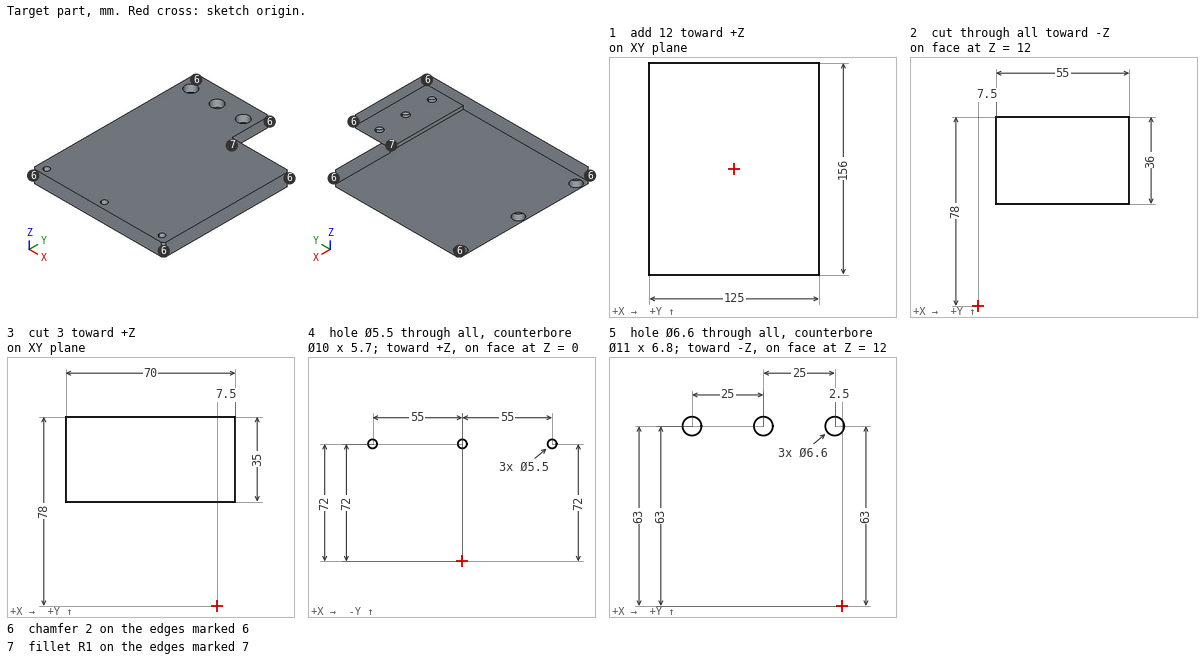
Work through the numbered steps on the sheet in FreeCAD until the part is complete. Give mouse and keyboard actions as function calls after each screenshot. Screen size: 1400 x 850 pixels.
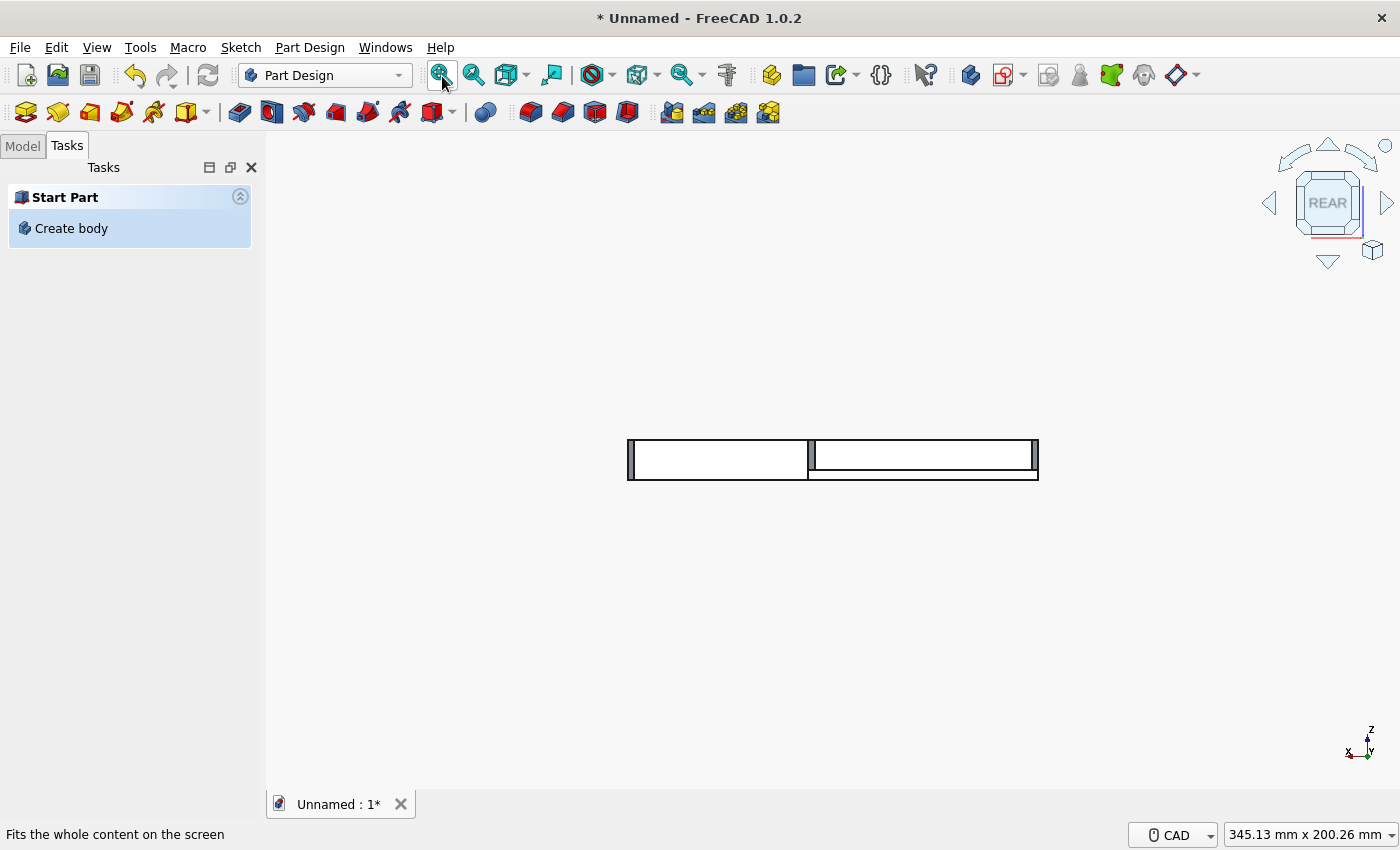
key(0)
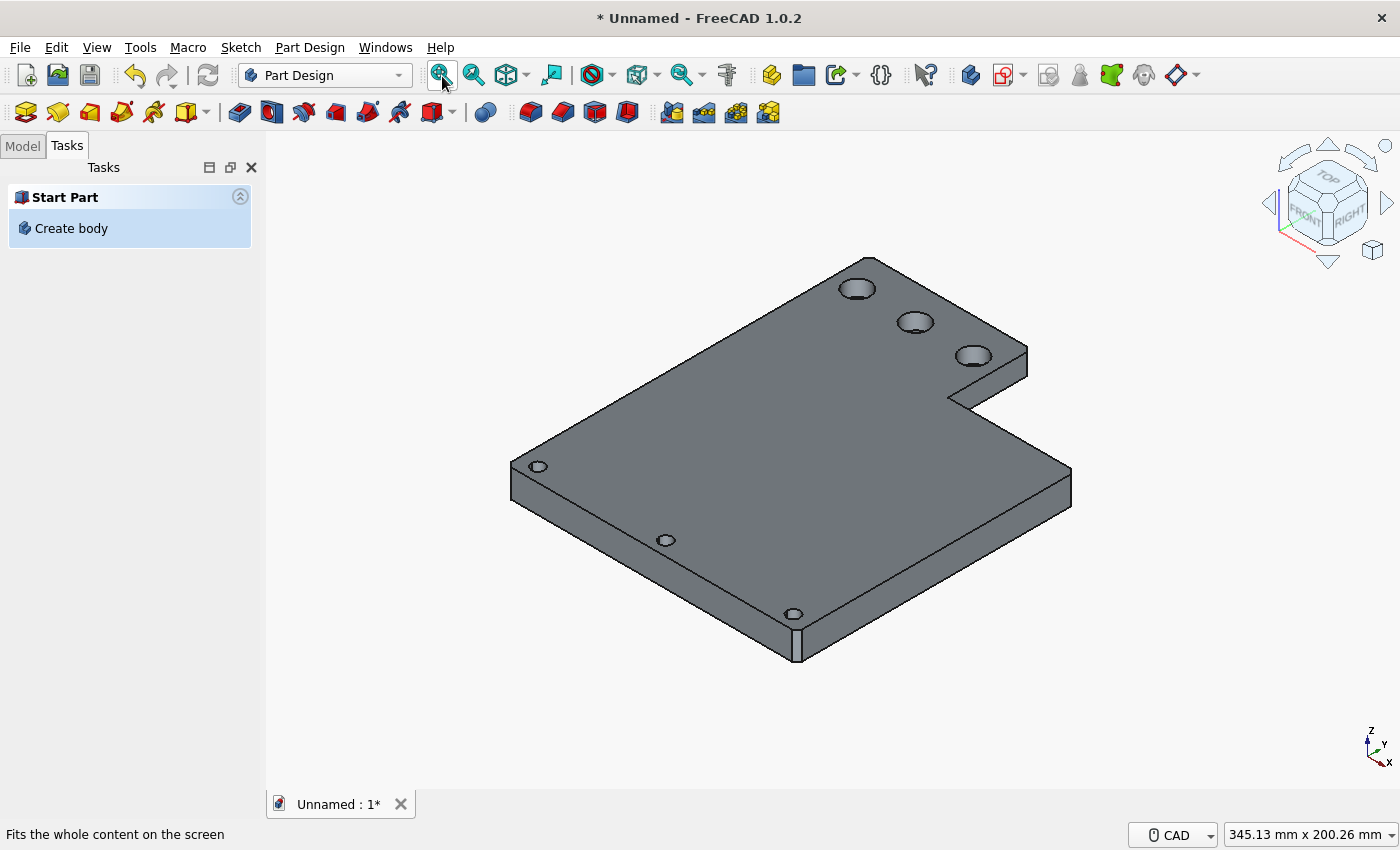
key(2)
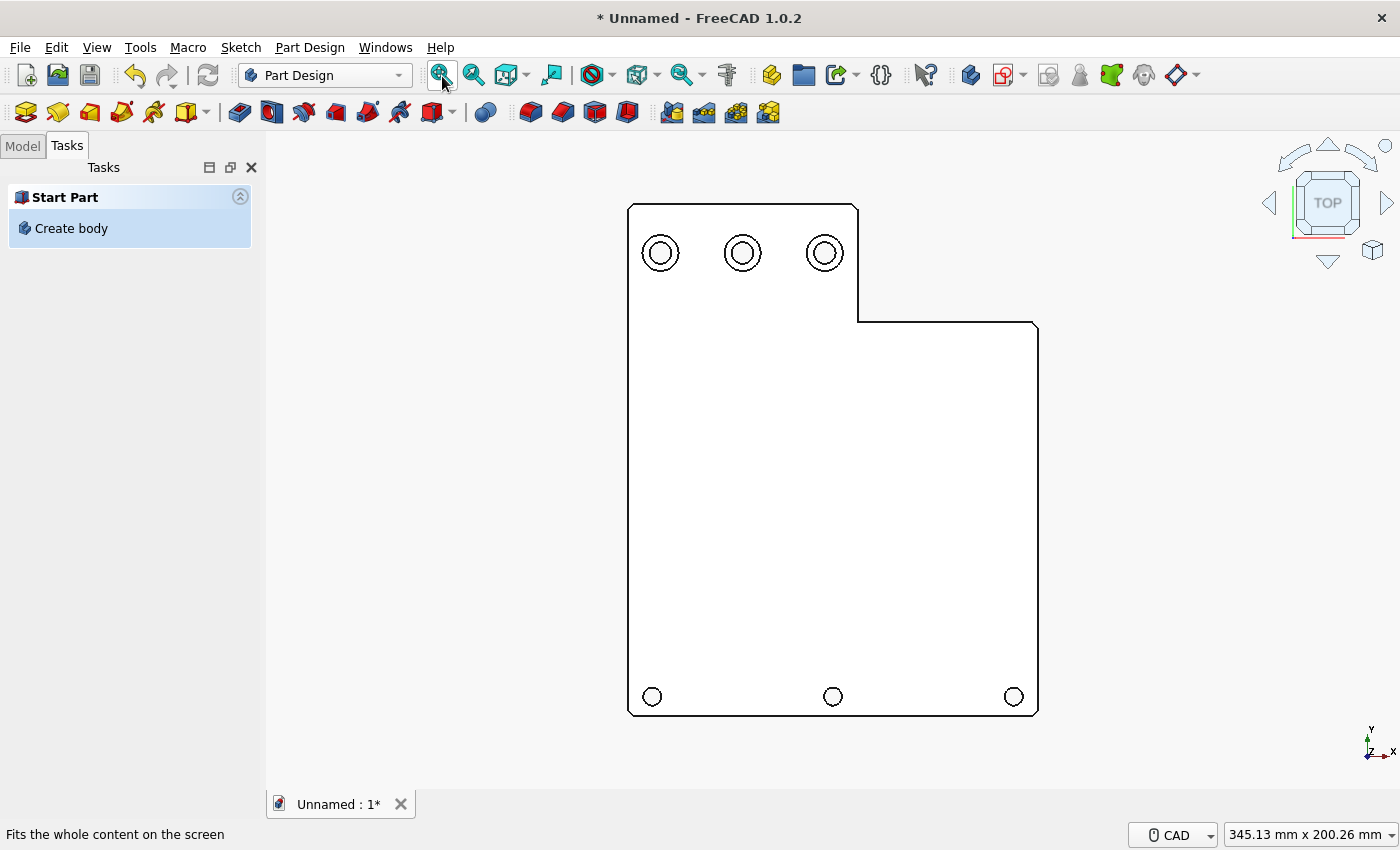
key(1)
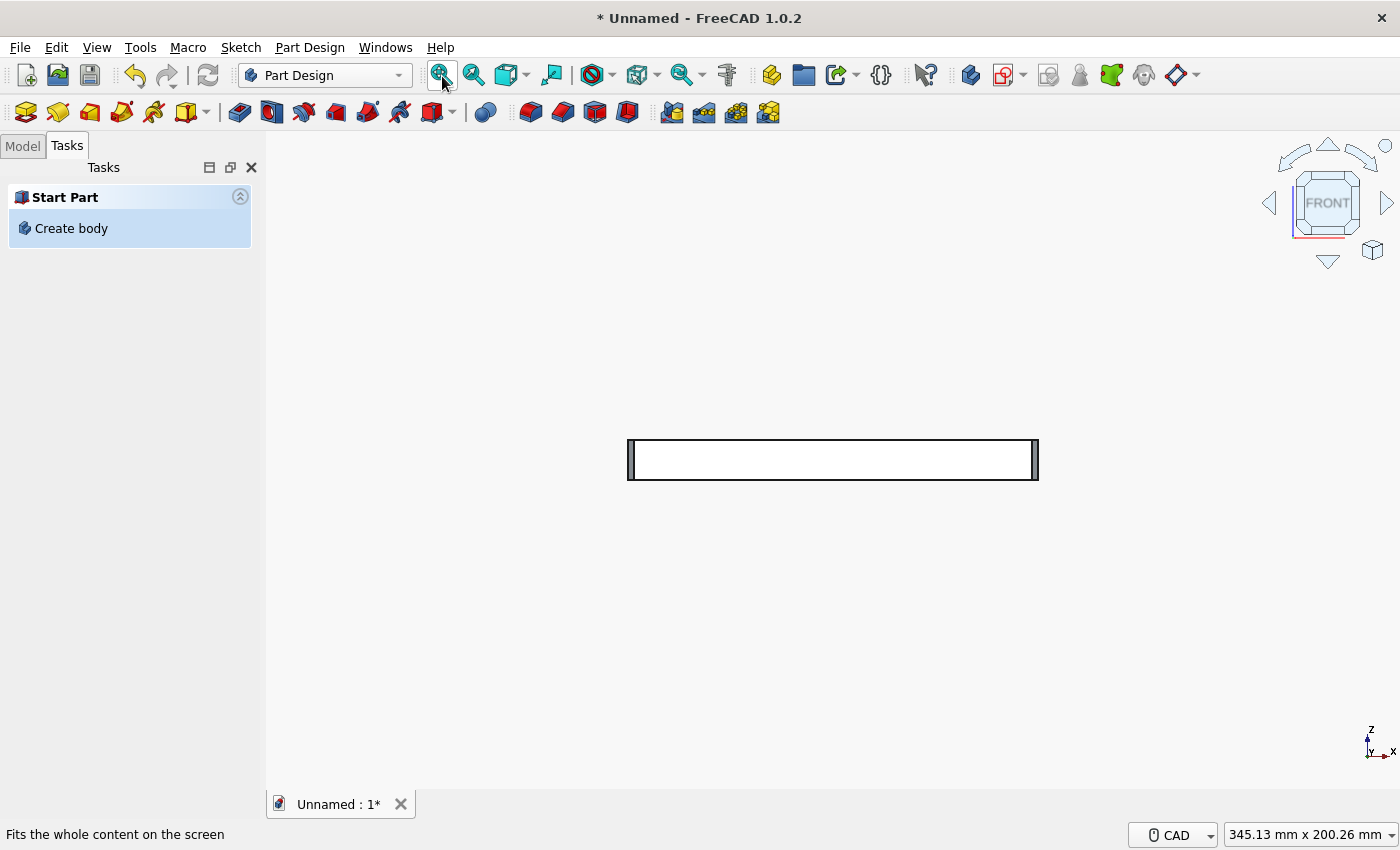
click(442, 76)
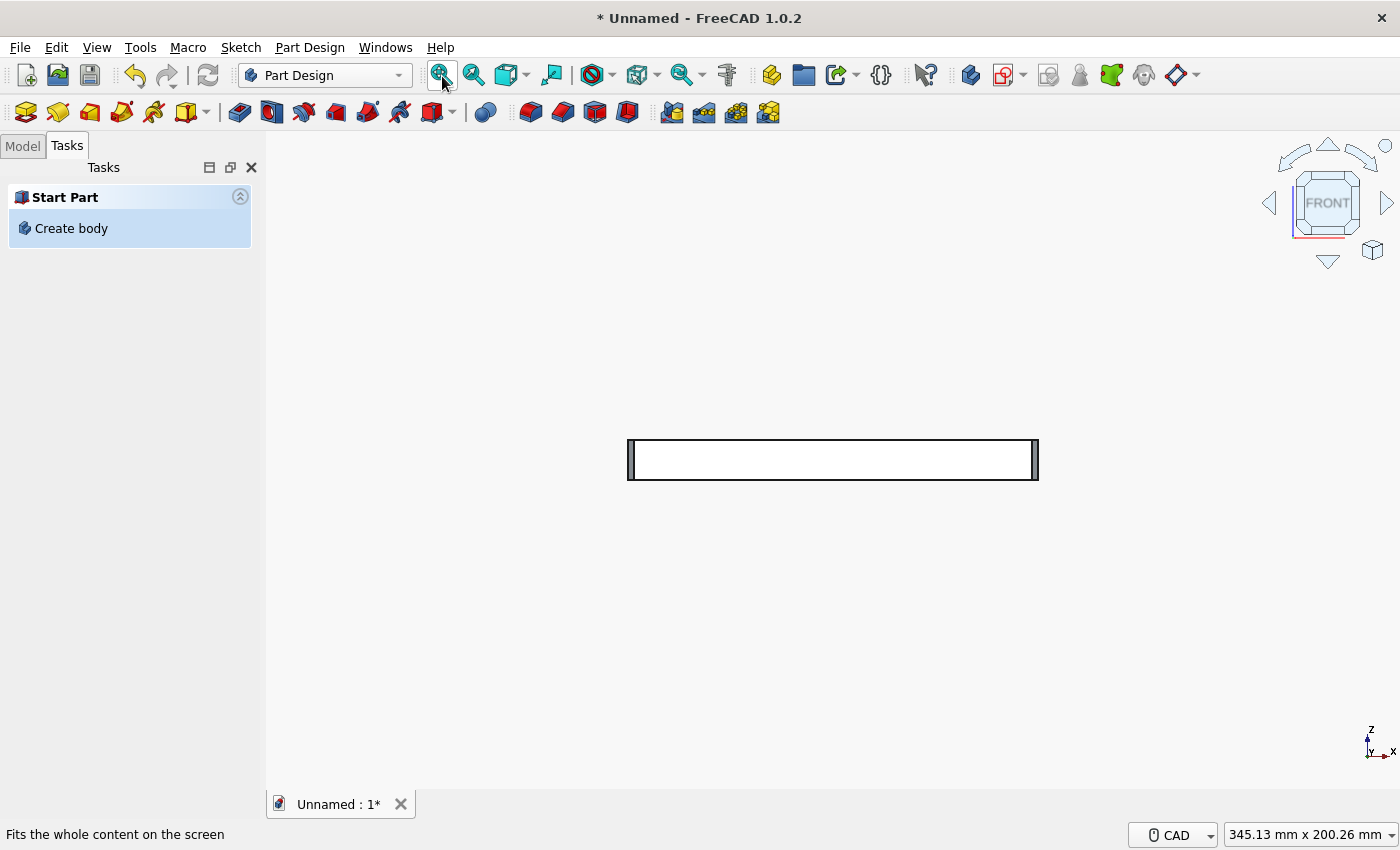
key(3)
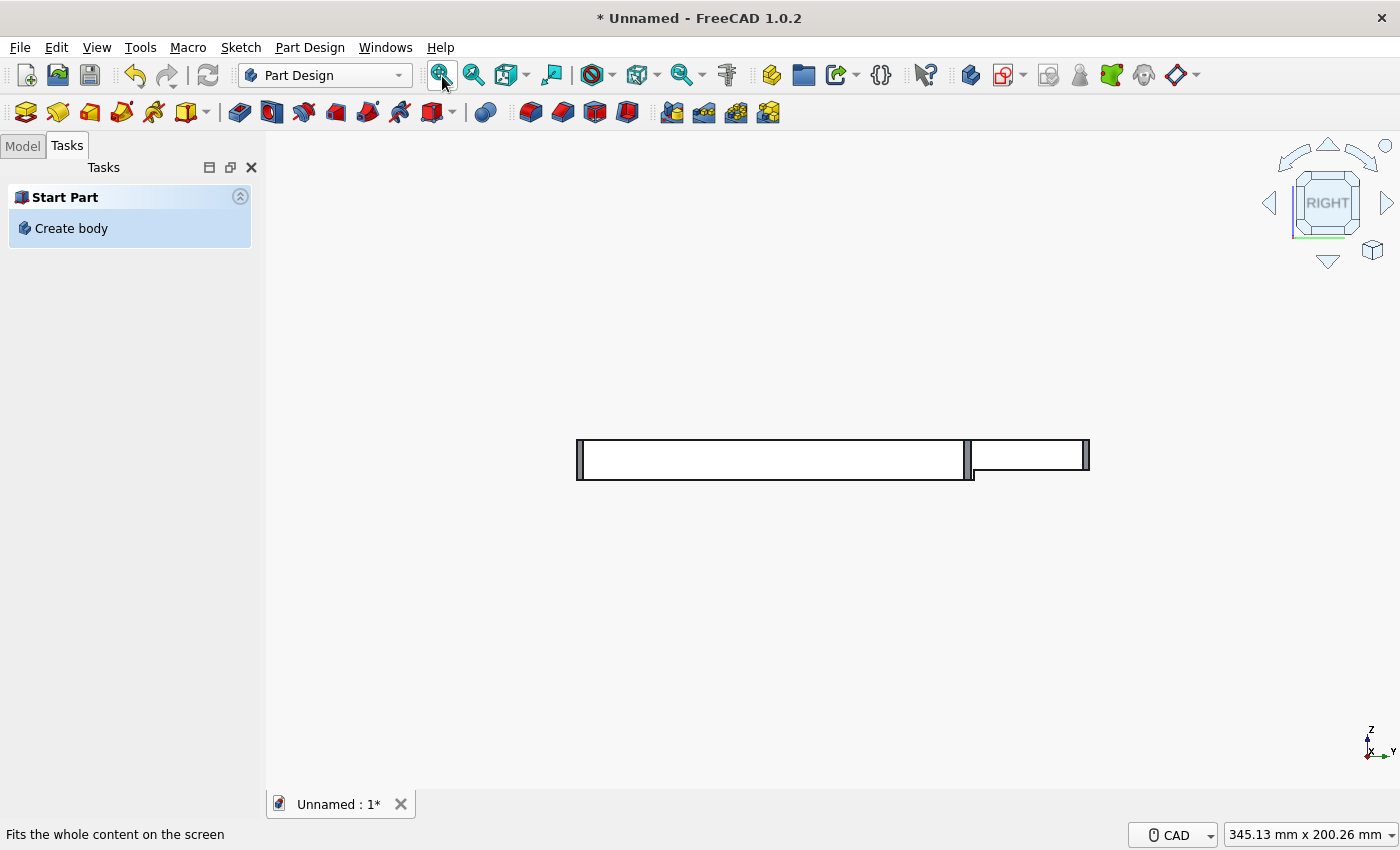
key(5)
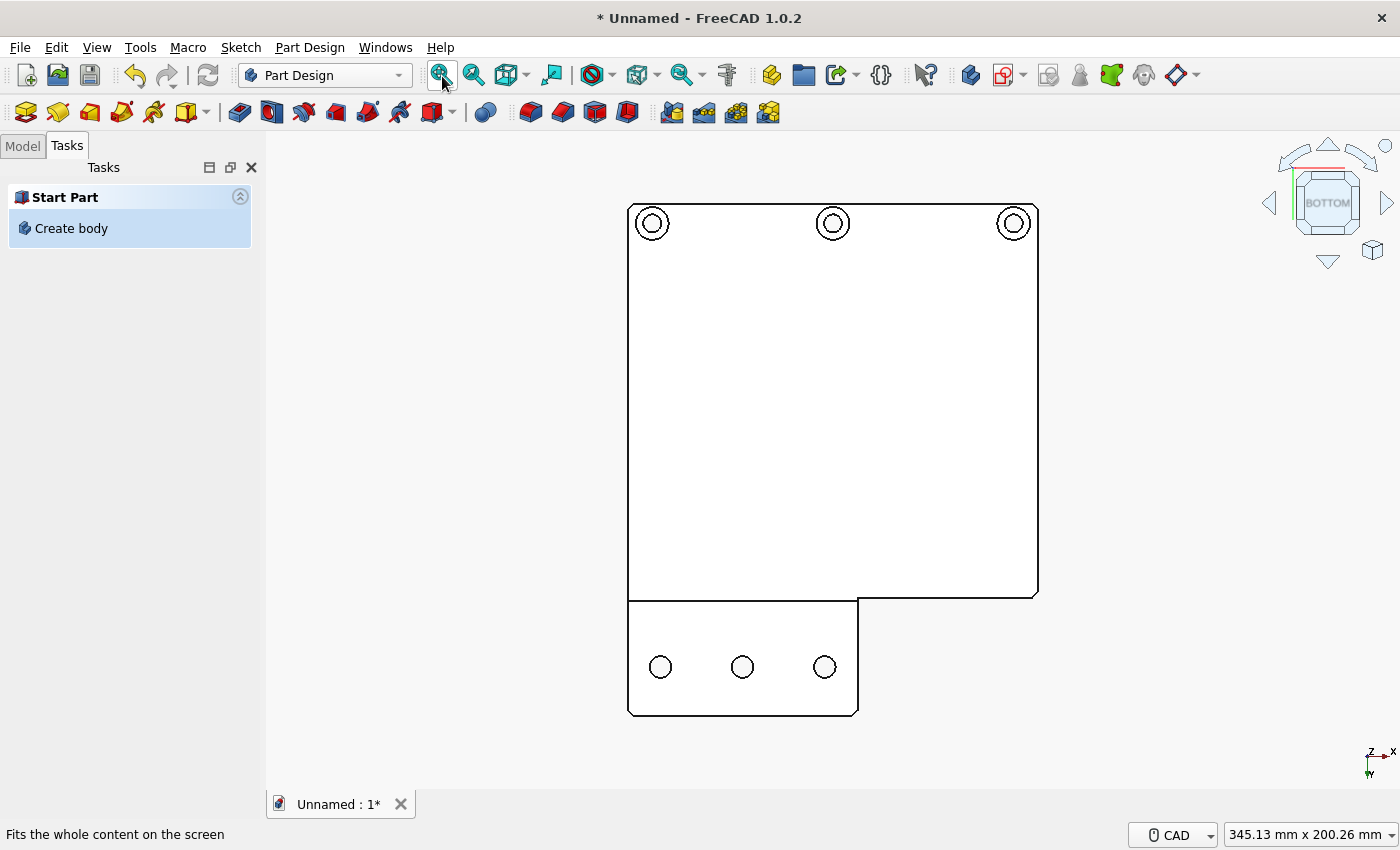
key(4)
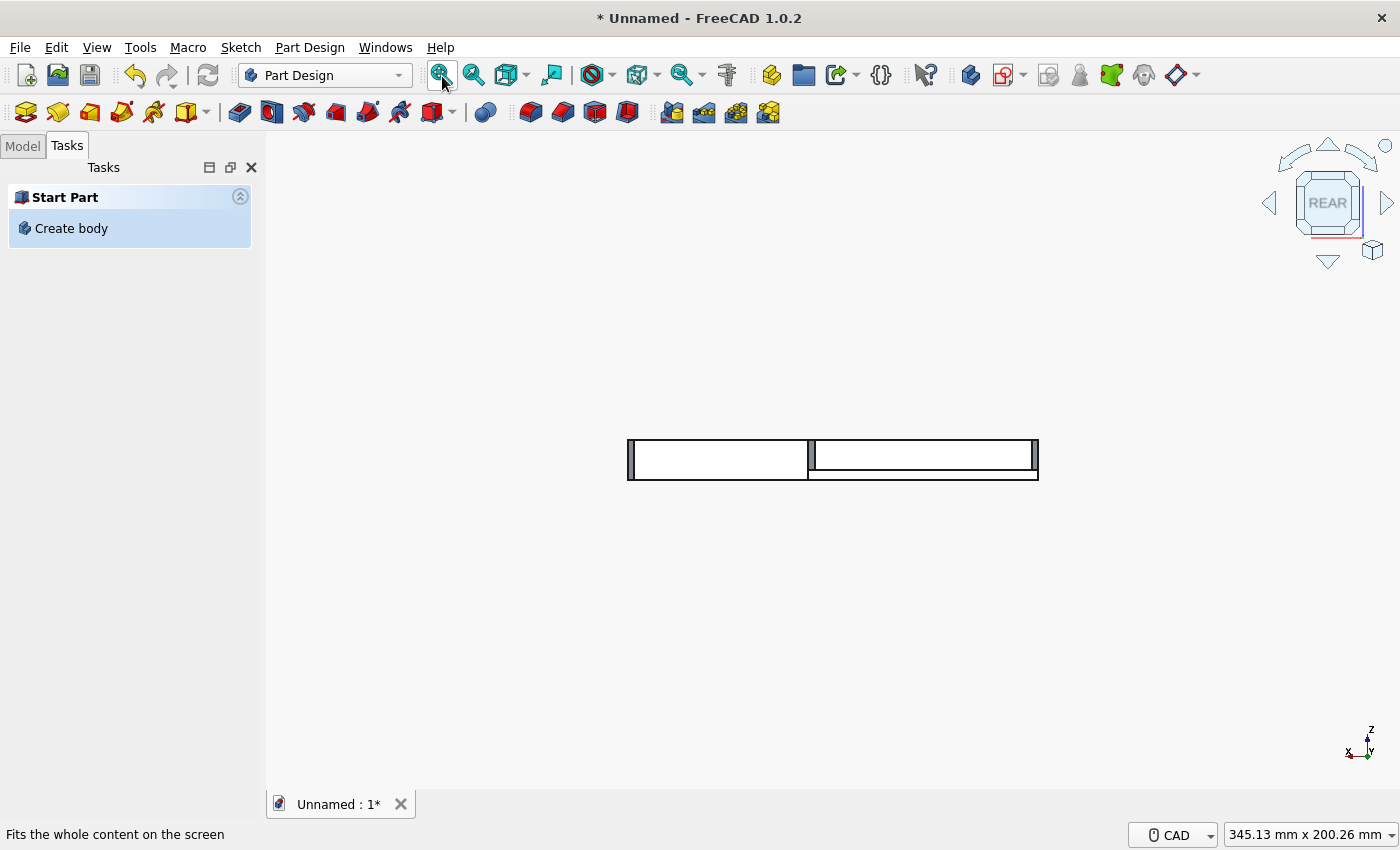
click(442, 76)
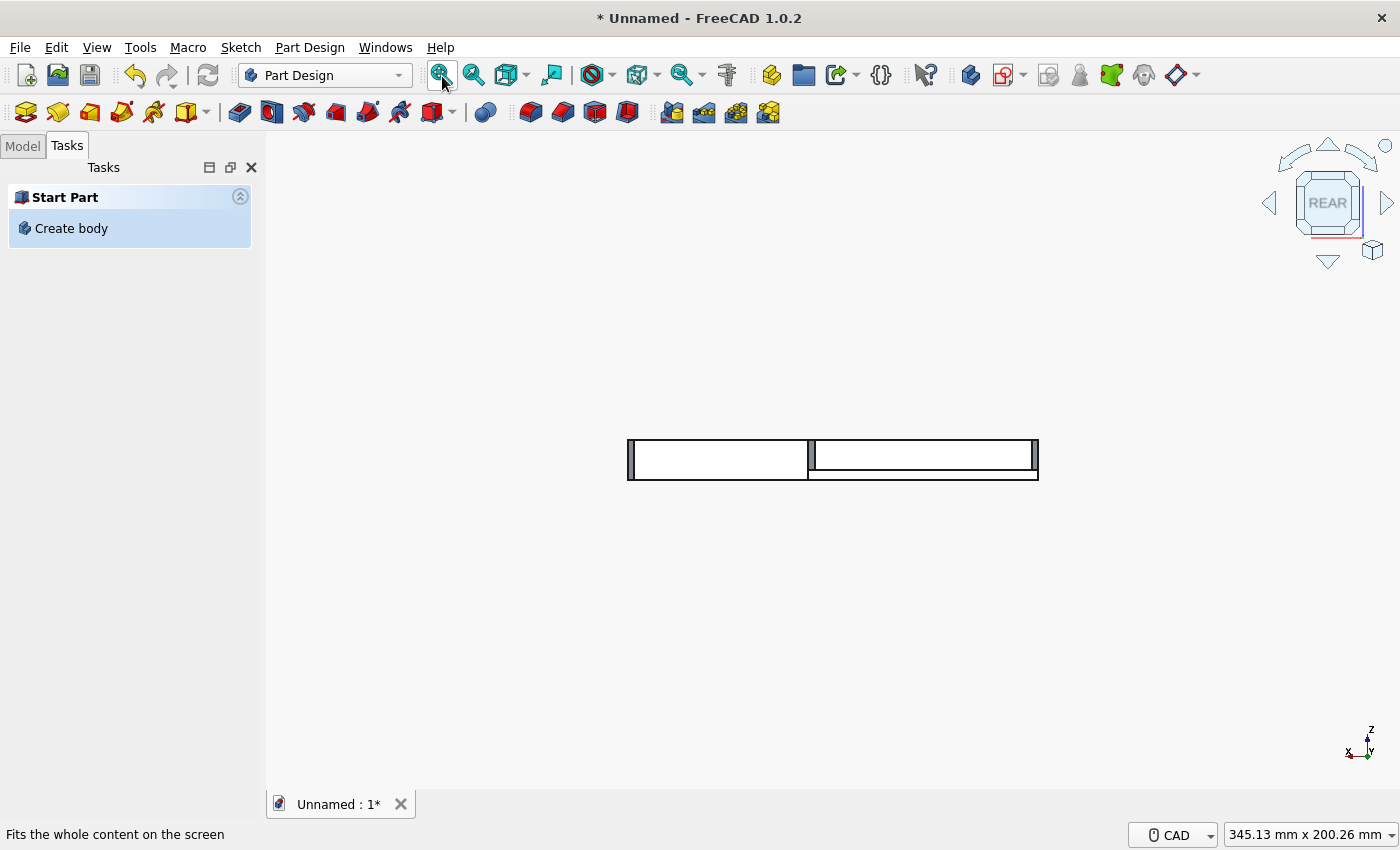
key(6)